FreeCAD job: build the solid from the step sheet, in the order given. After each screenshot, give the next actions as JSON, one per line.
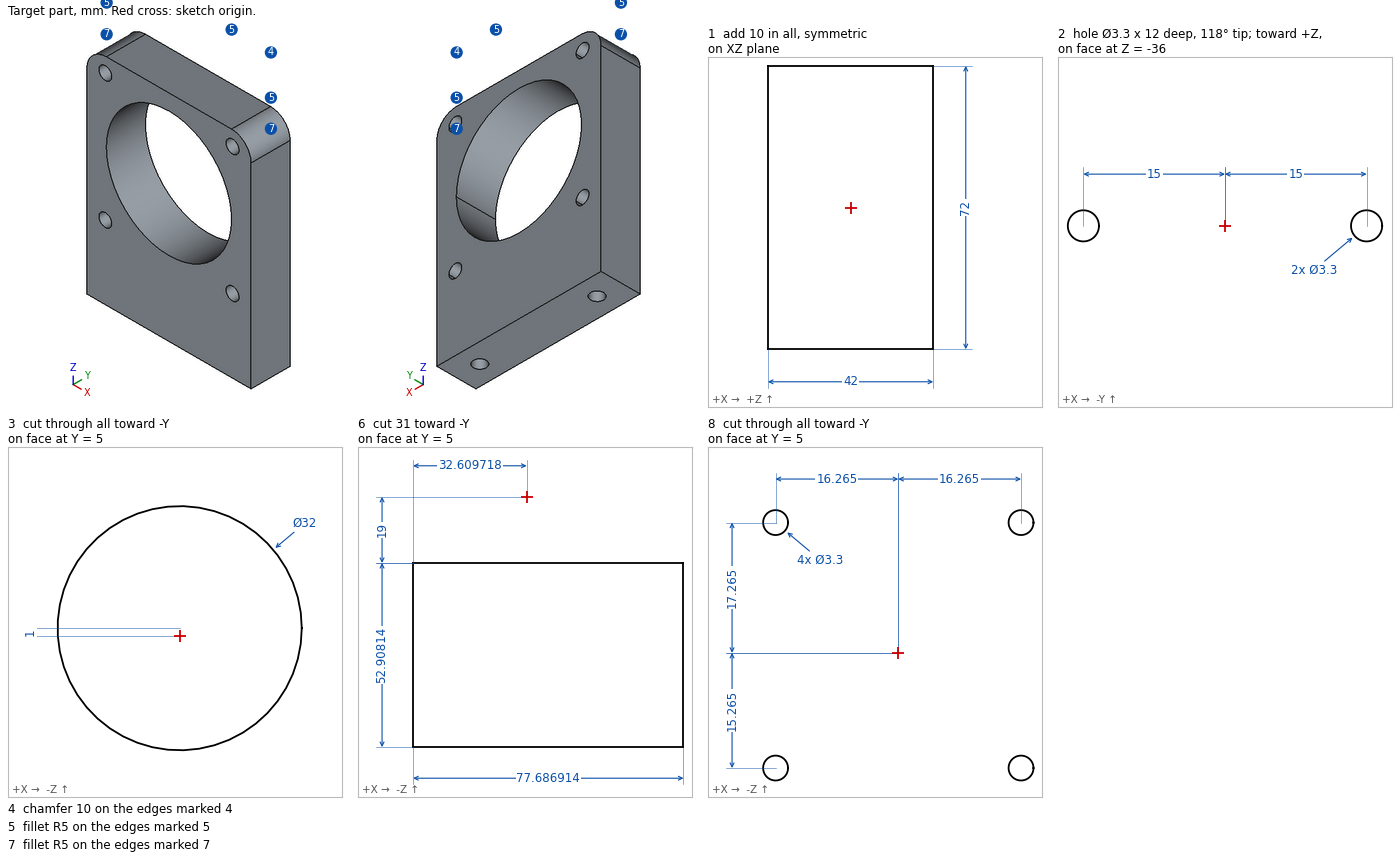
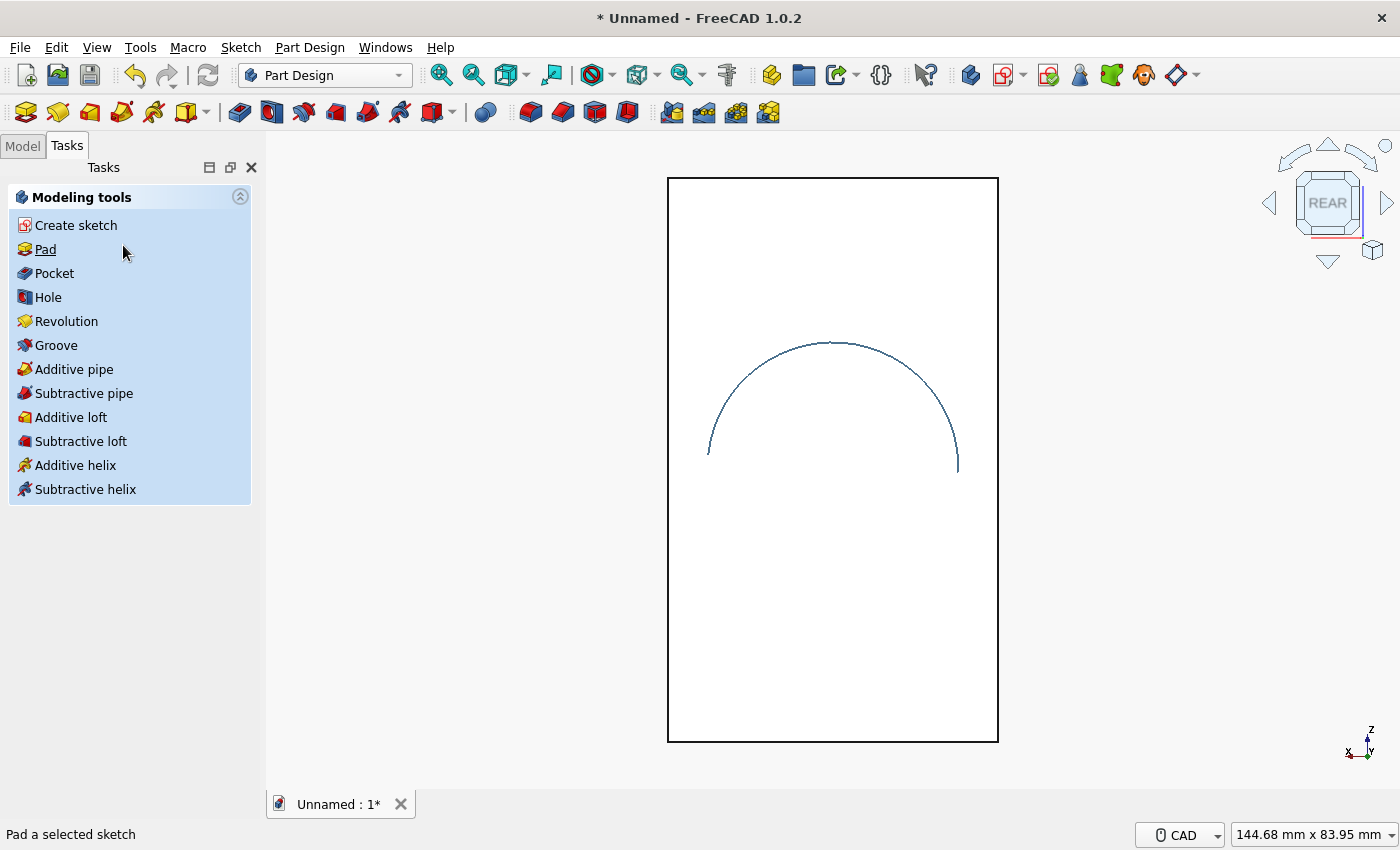
{"action": "left_click", "coordinate": [240, 112]}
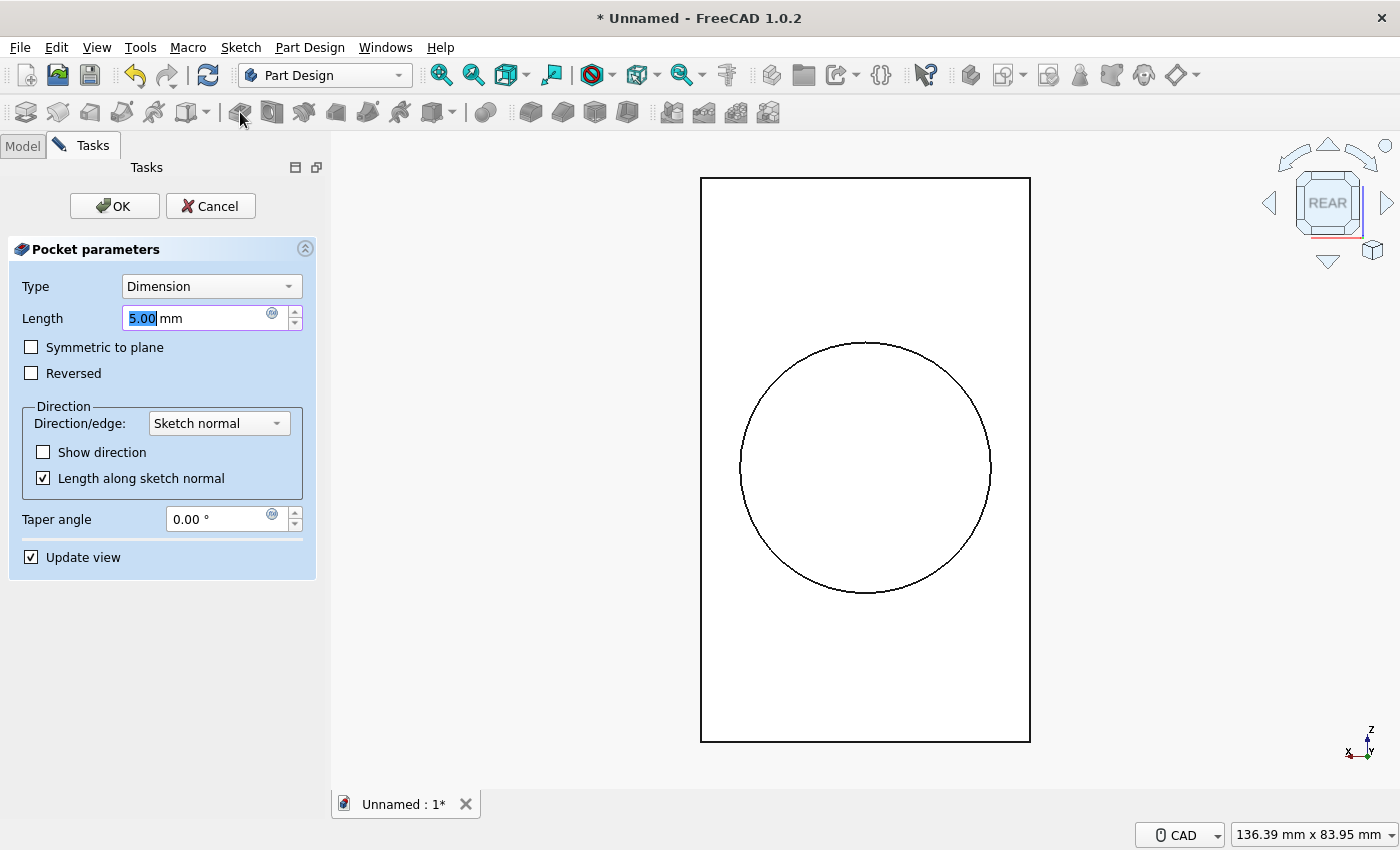
{"action": "left_click", "coordinate": [212, 286]}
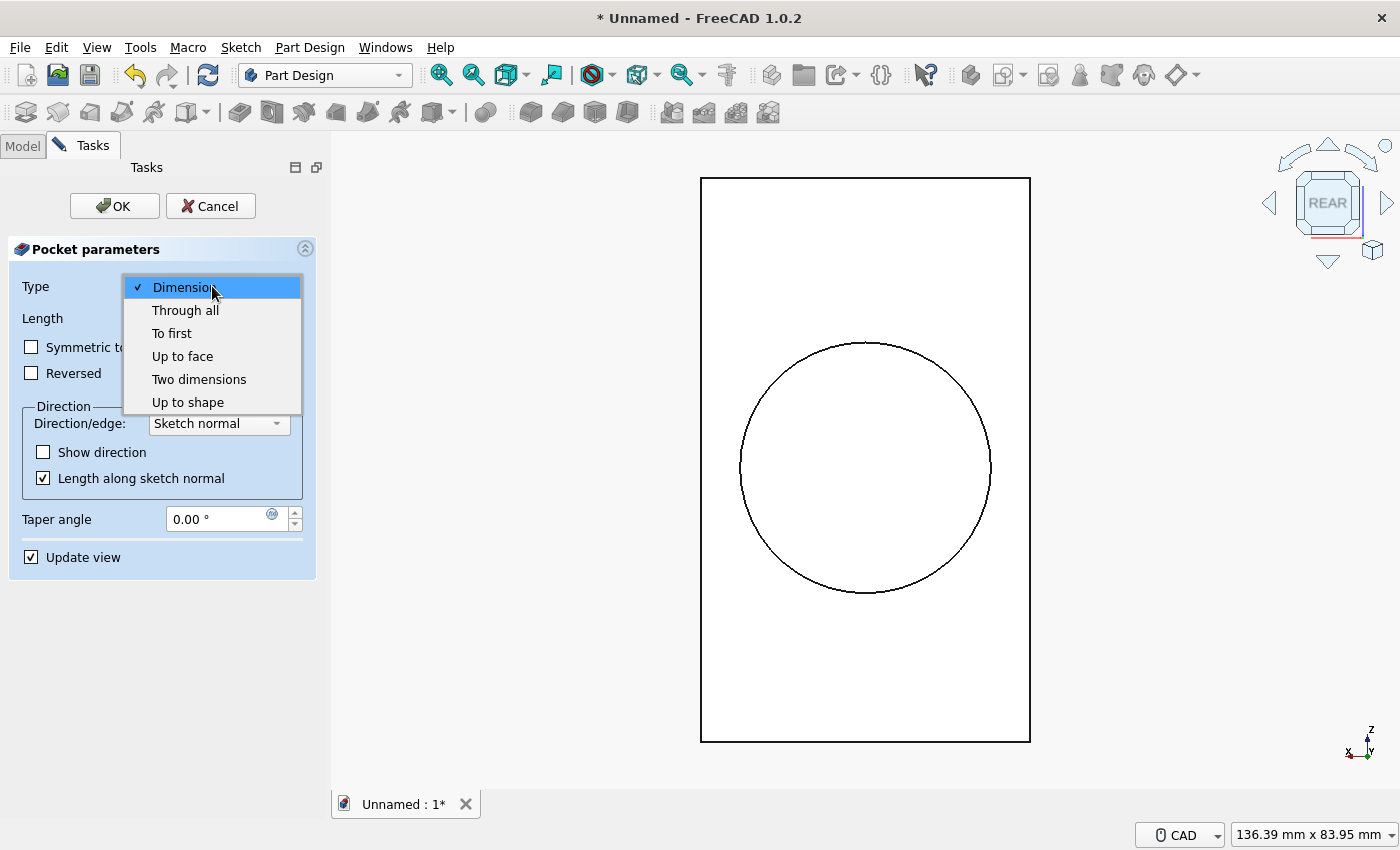
{"action": "left_click", "coordinate": [212, 310]}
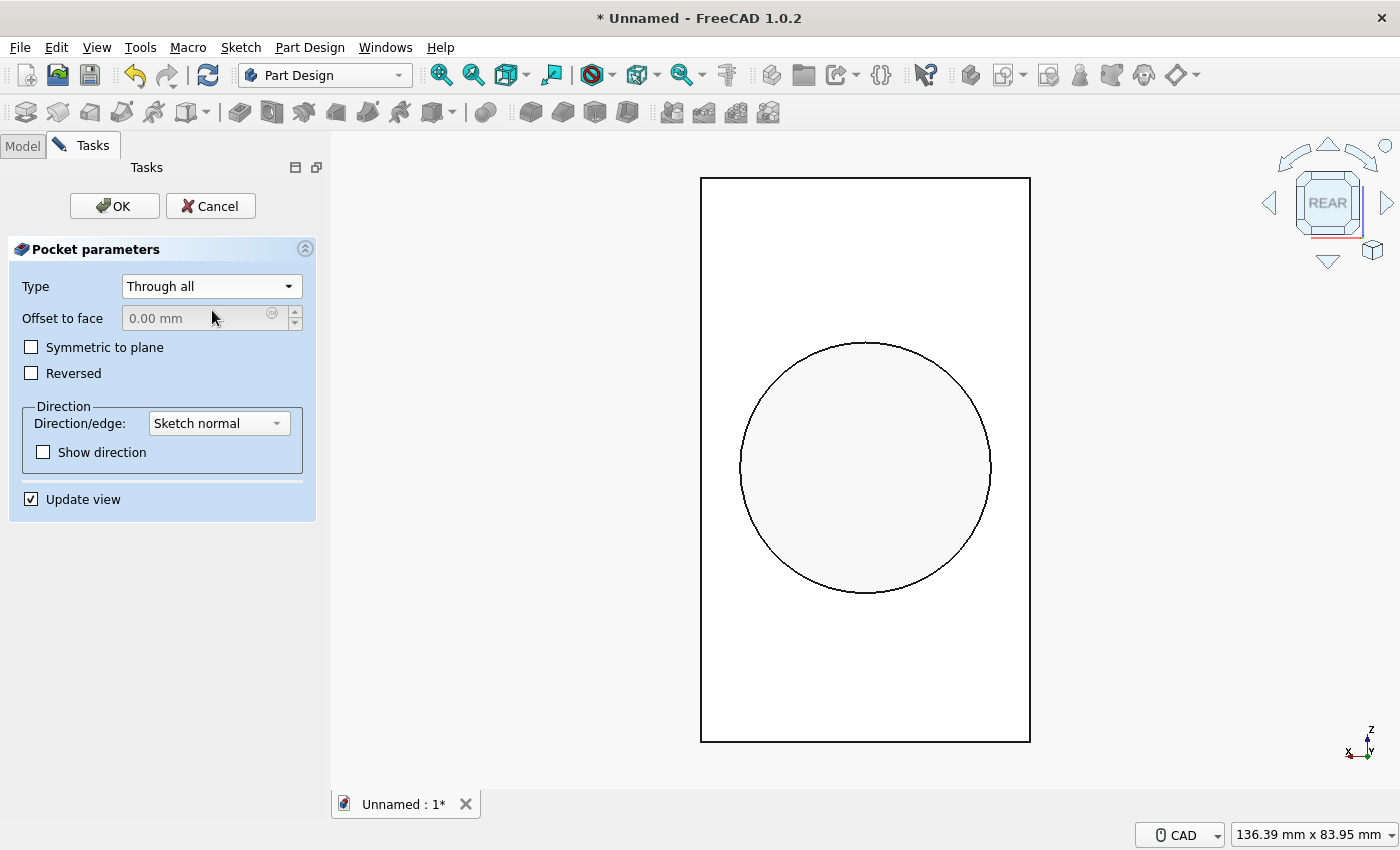
{"action": "left_click", "coordinate": [115, 206]}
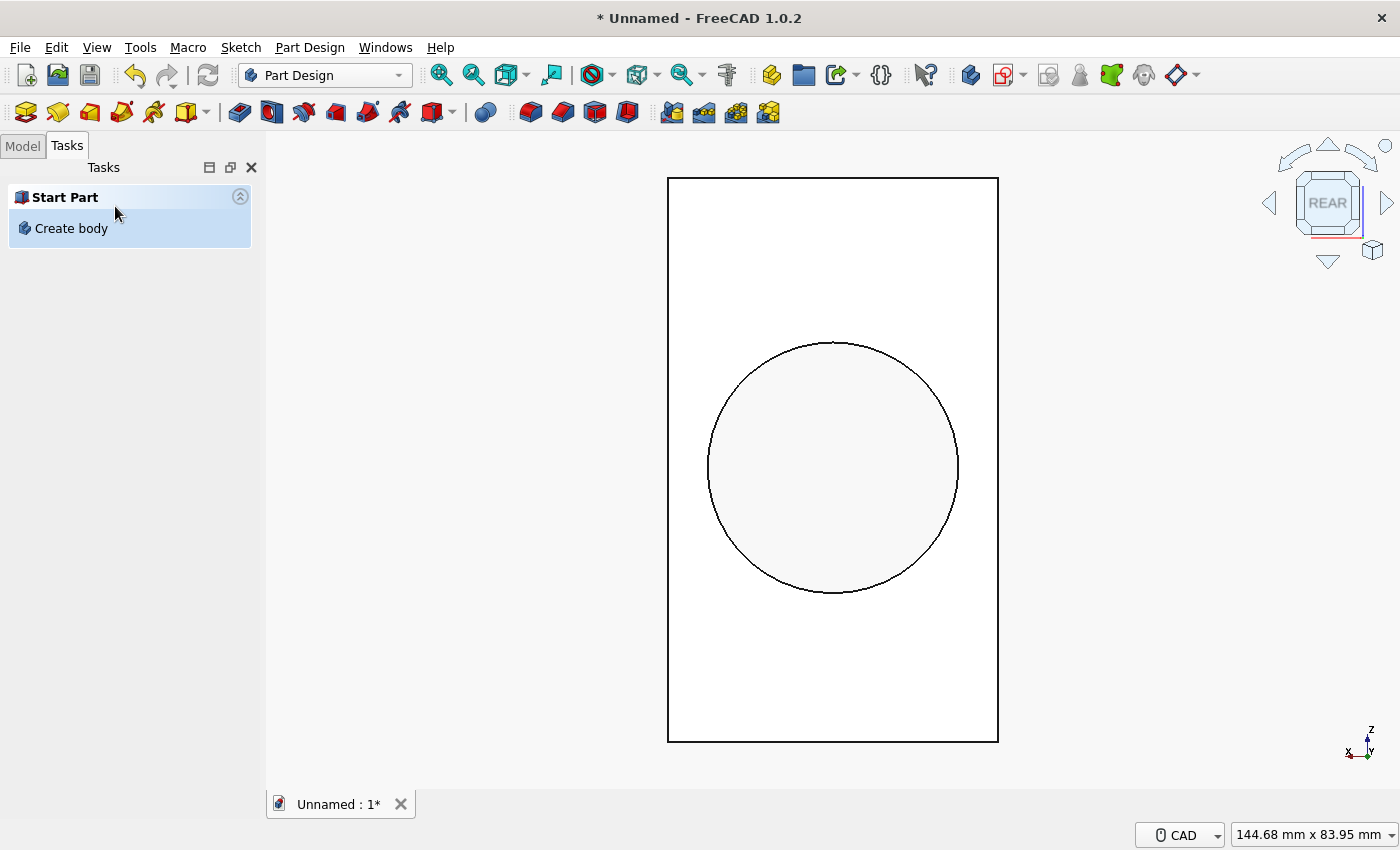
{"action": "key", "text": "0"}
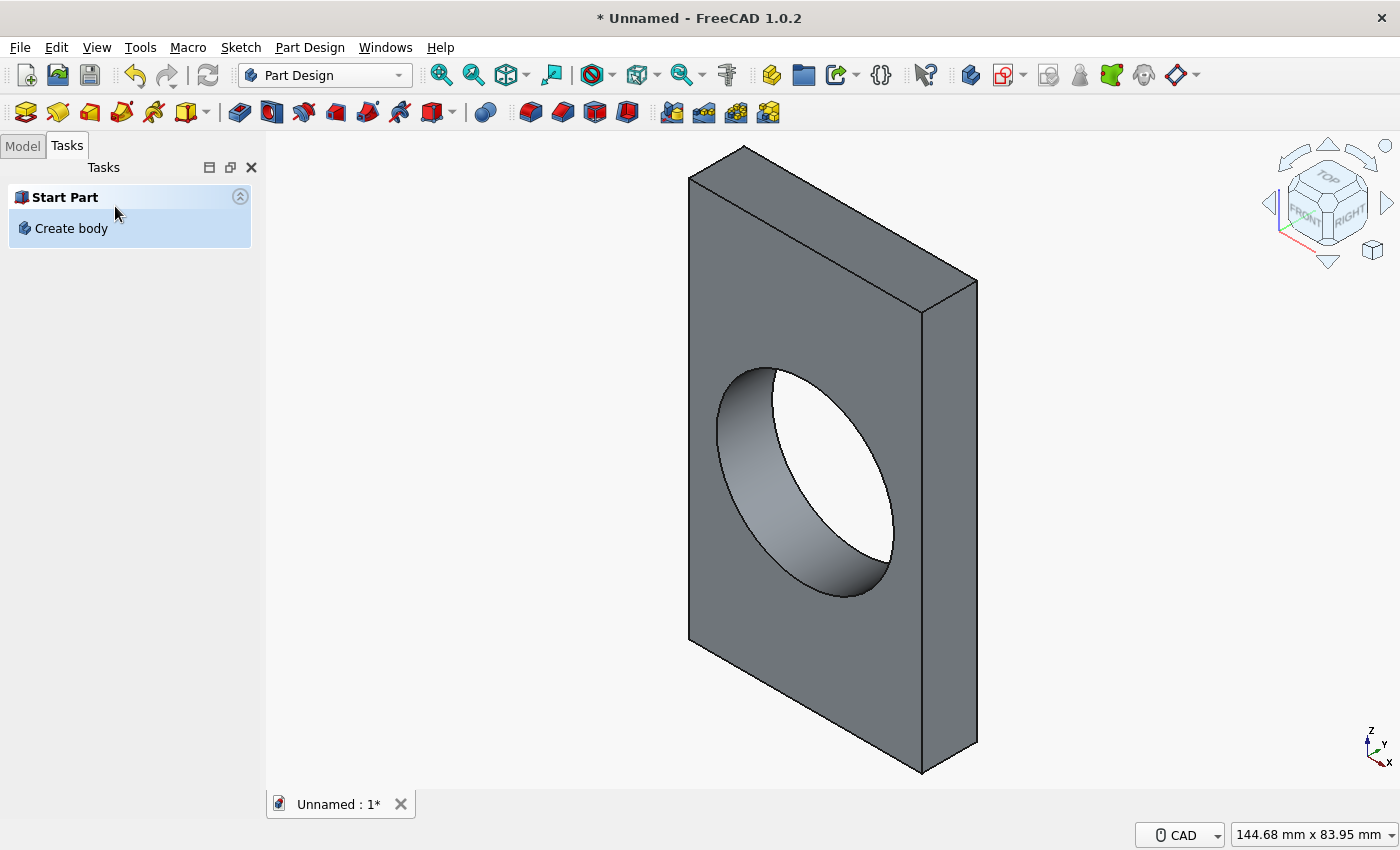
{"action": "left_click", "coordinate": [949, 296]}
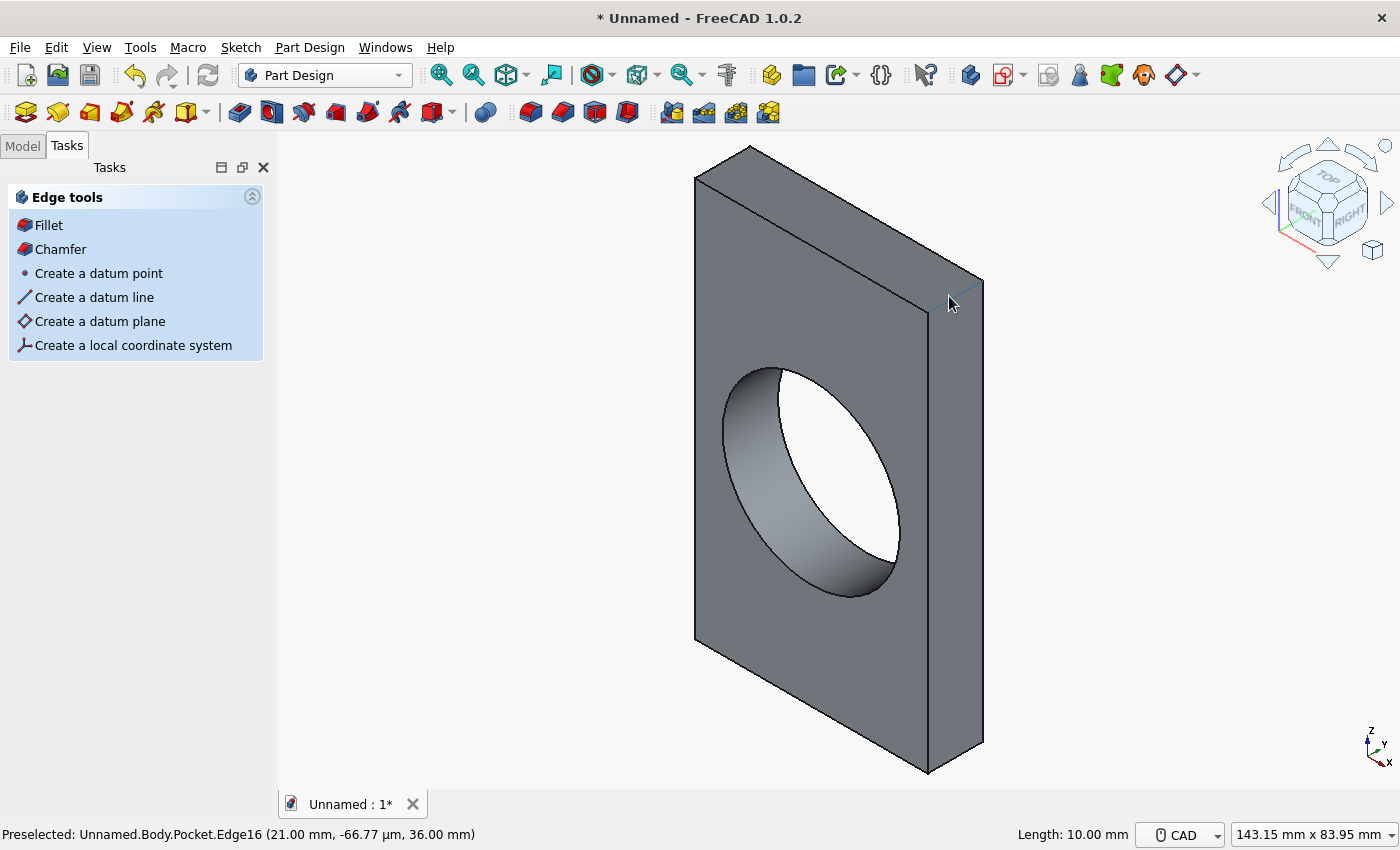
{"action": "key", "text": "2"}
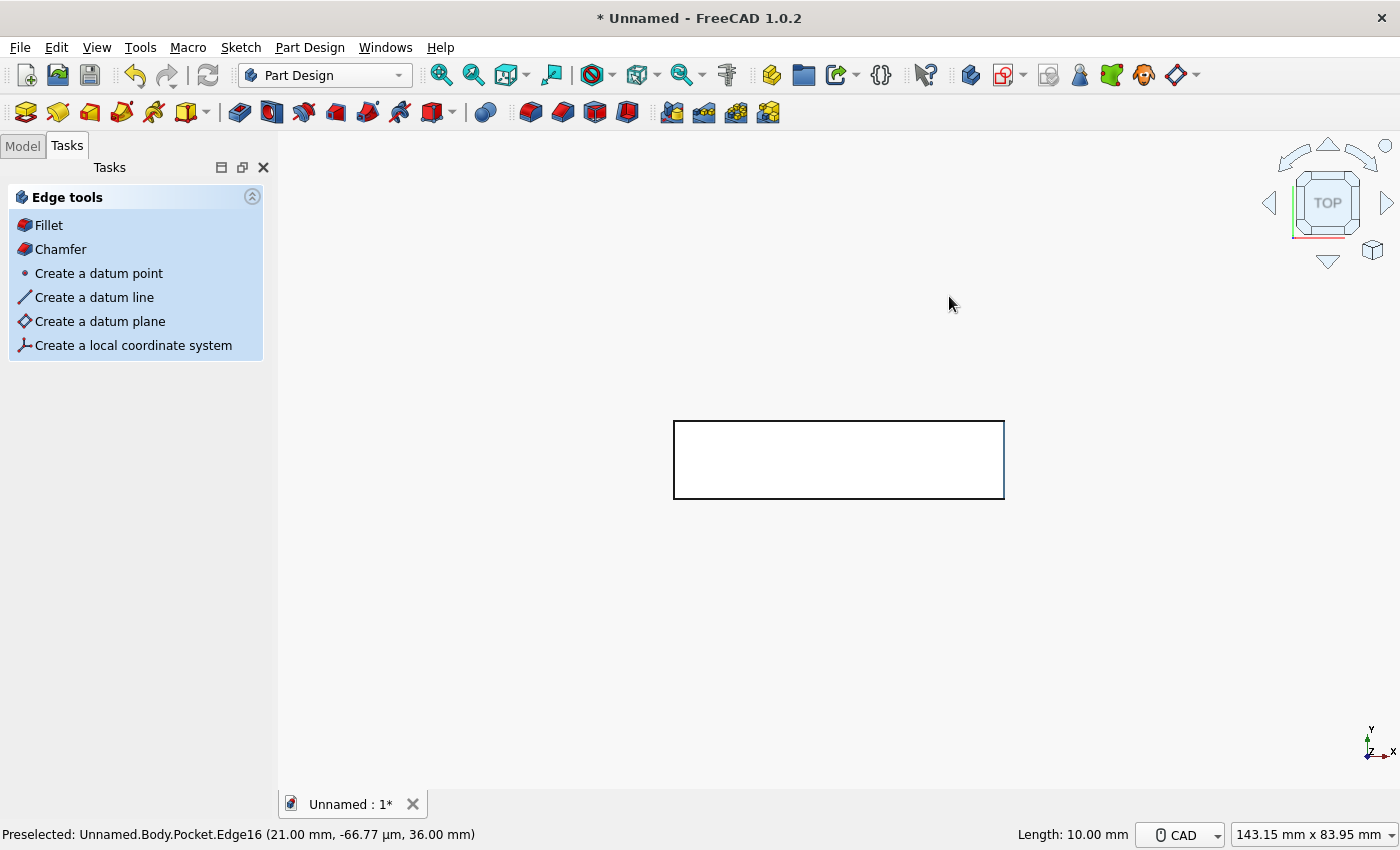
{"action": "left_click", "coordinate": [442, 76]}